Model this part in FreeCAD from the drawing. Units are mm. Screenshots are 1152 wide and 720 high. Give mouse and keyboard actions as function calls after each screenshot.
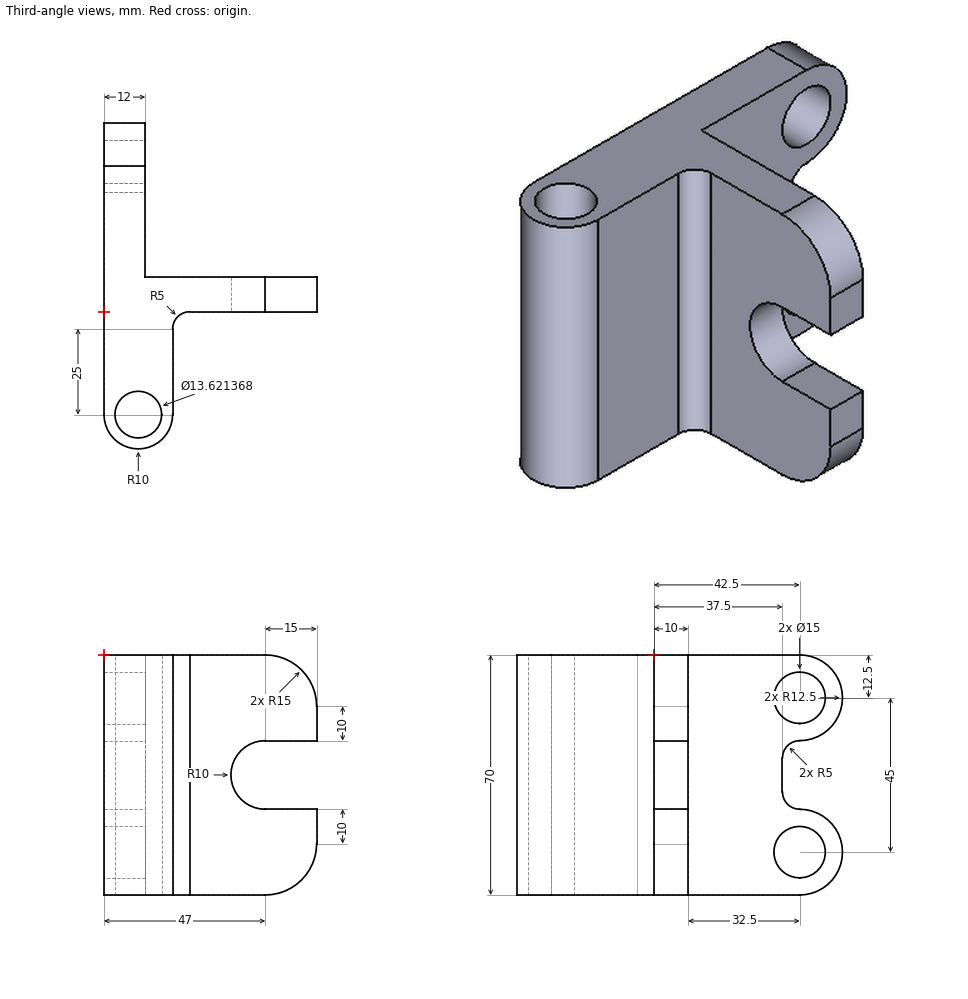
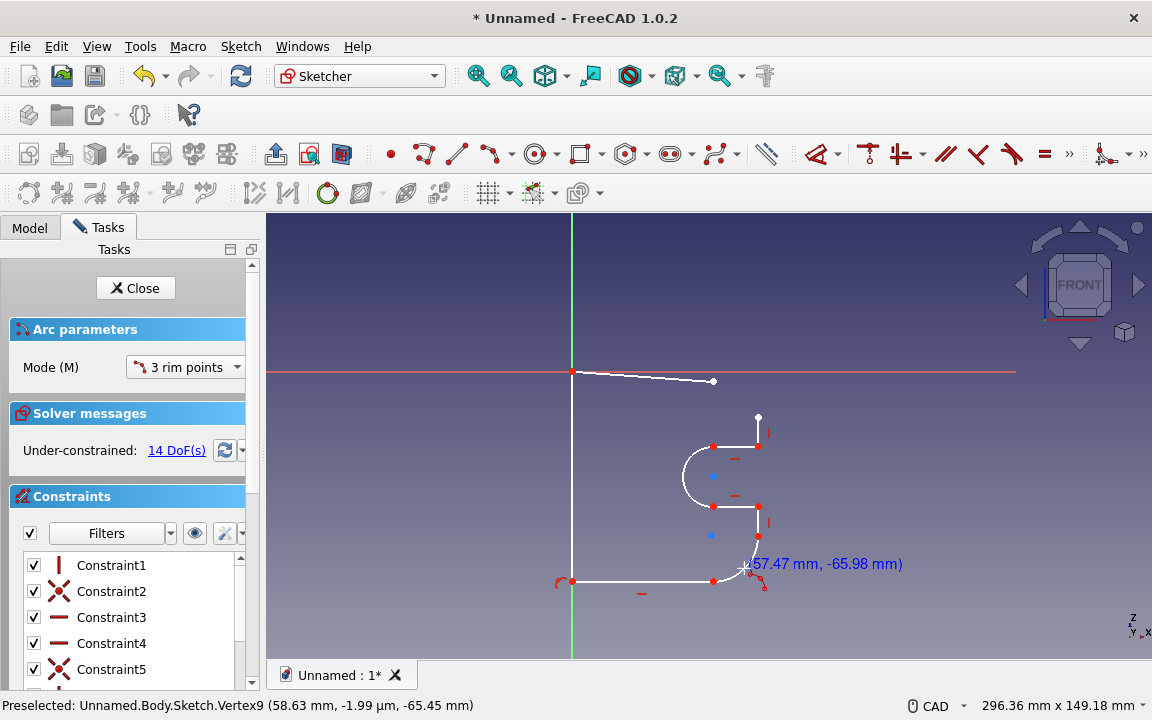
click(713, 382)
click(758, 418)
click(744, 385)
key(Escape)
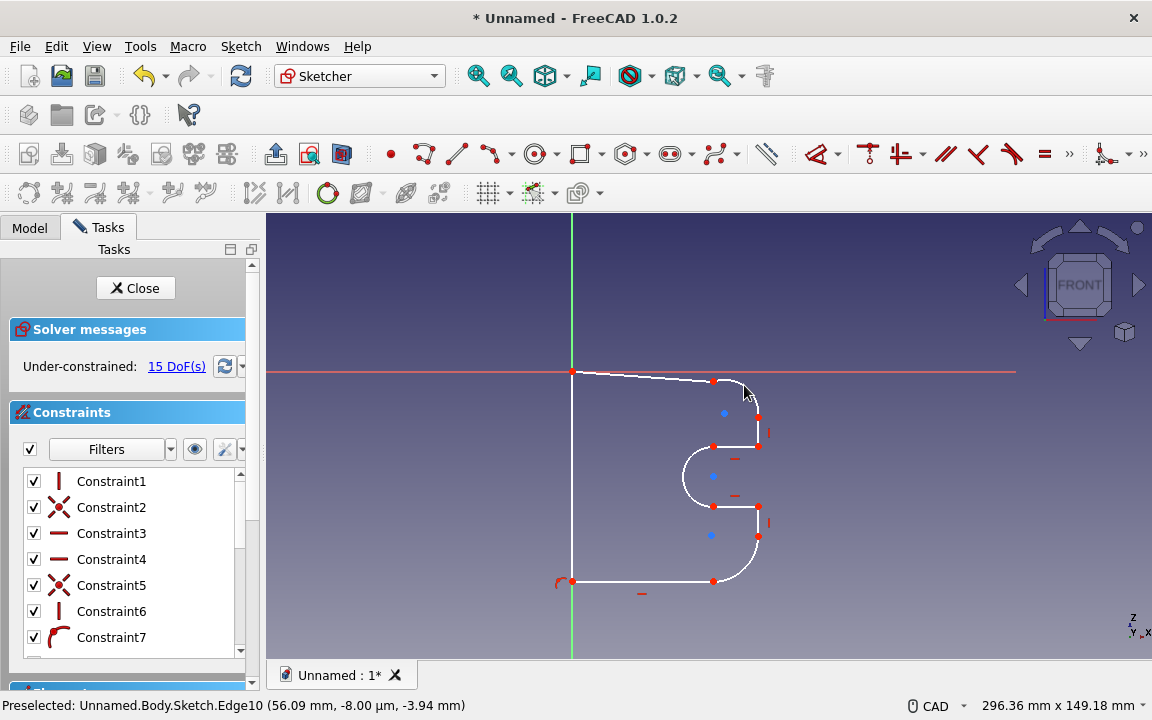
click(758, 430)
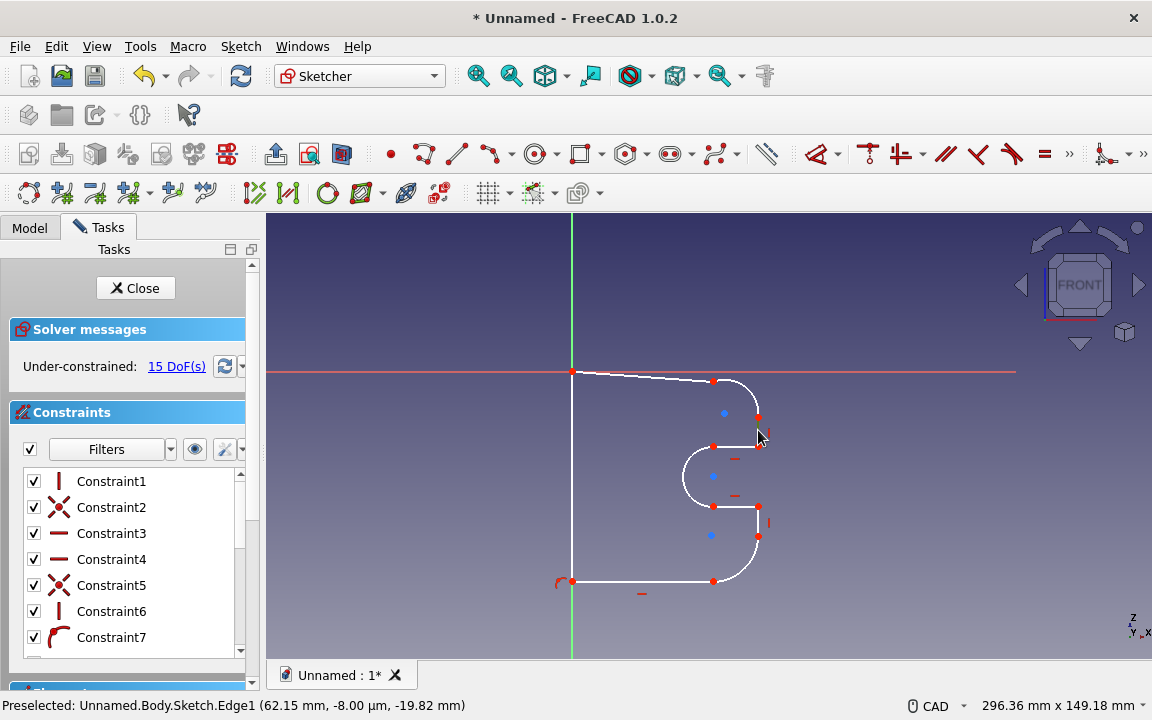
click(754, 398)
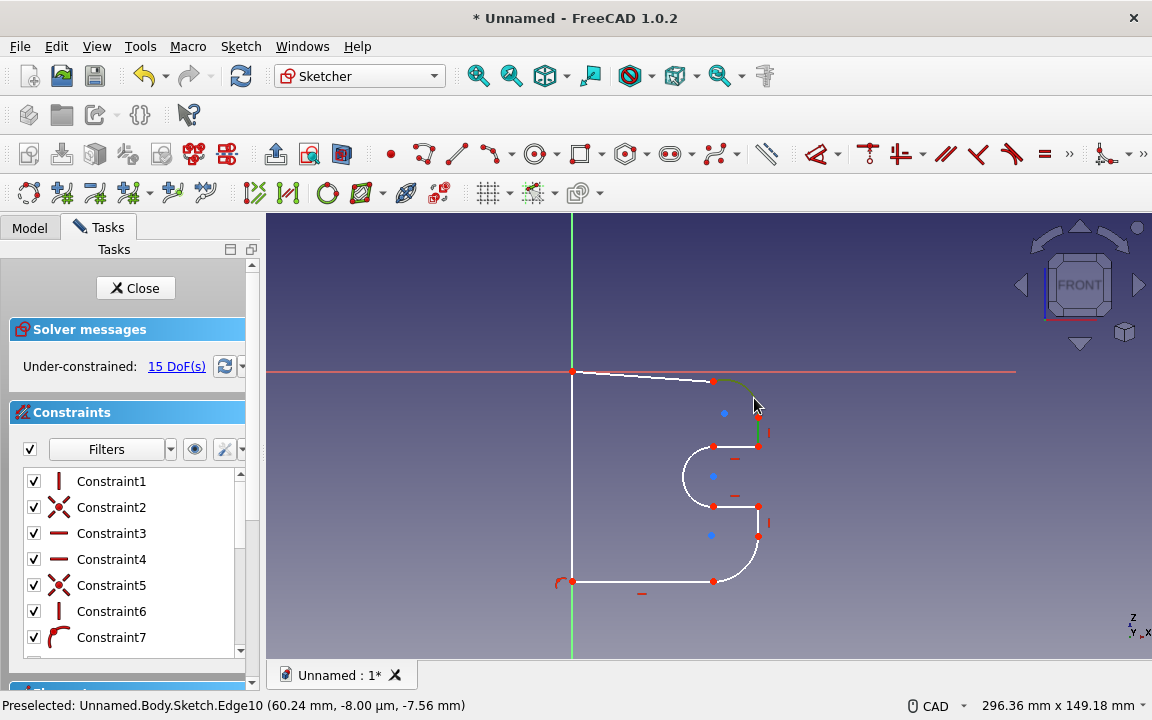
key(t)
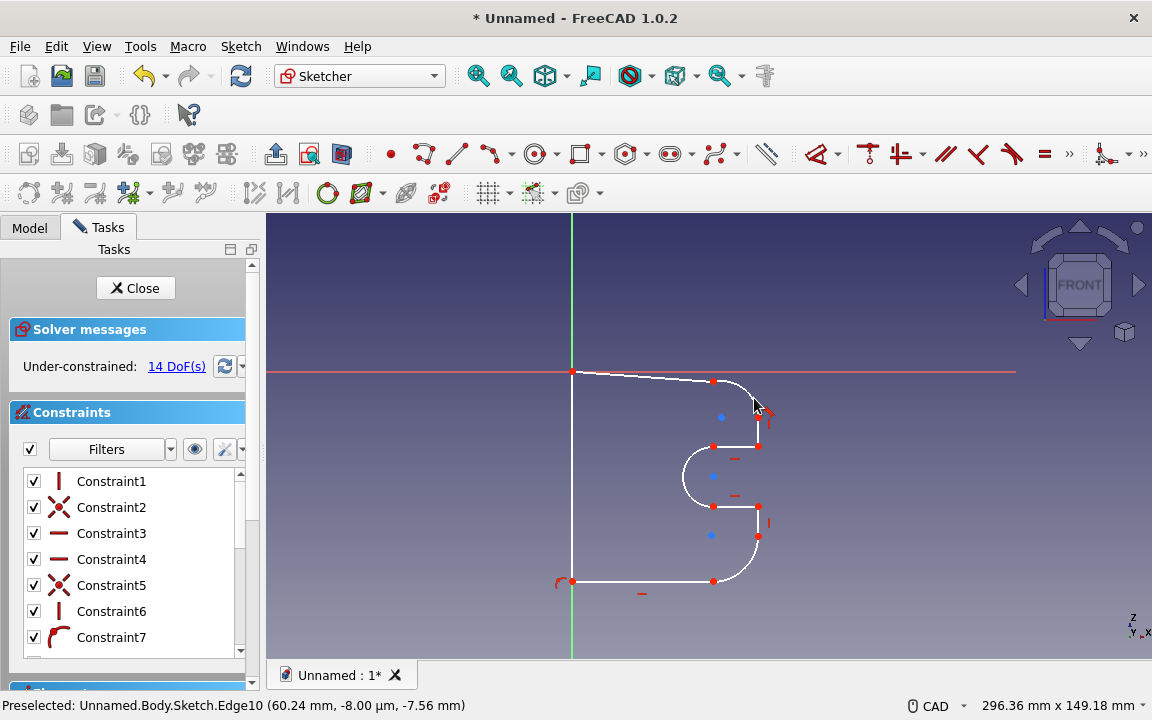
click(745, 447)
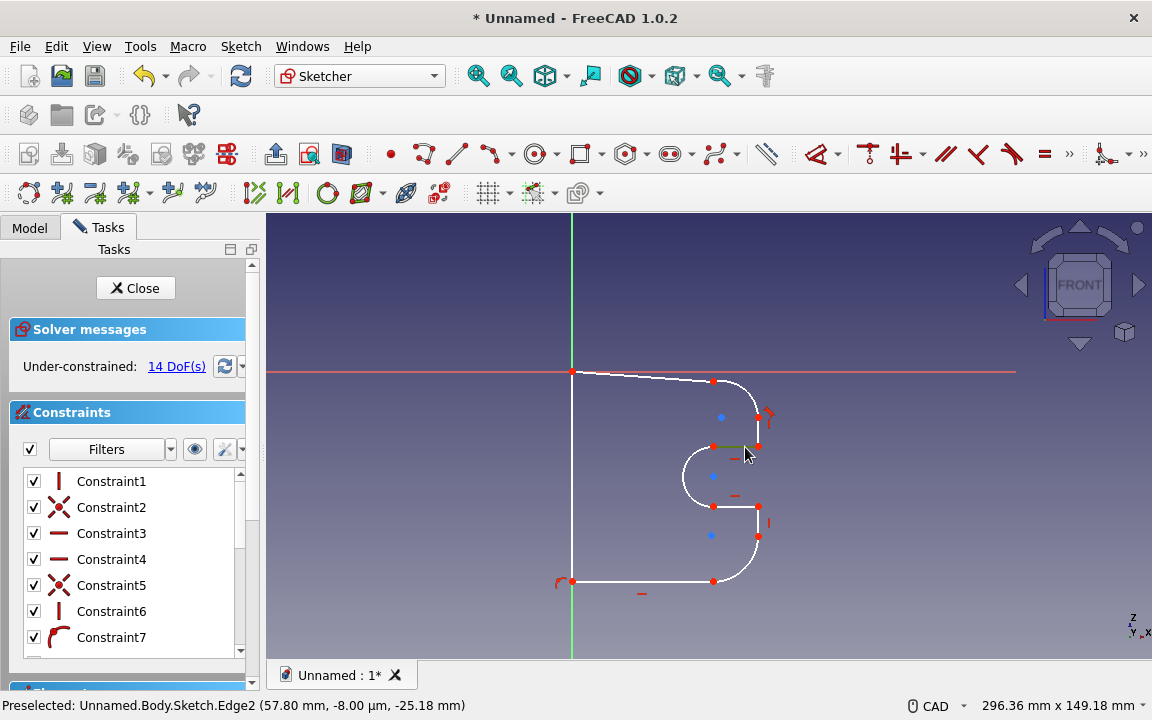
click(689, 459)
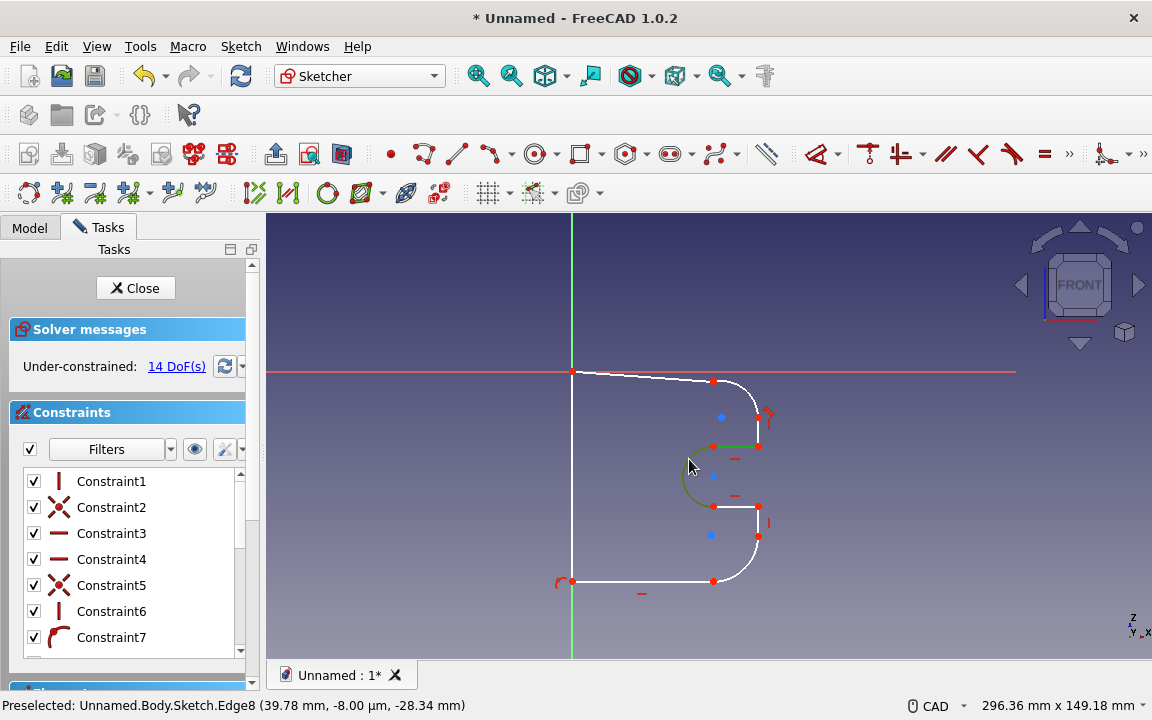
click(1012, 154)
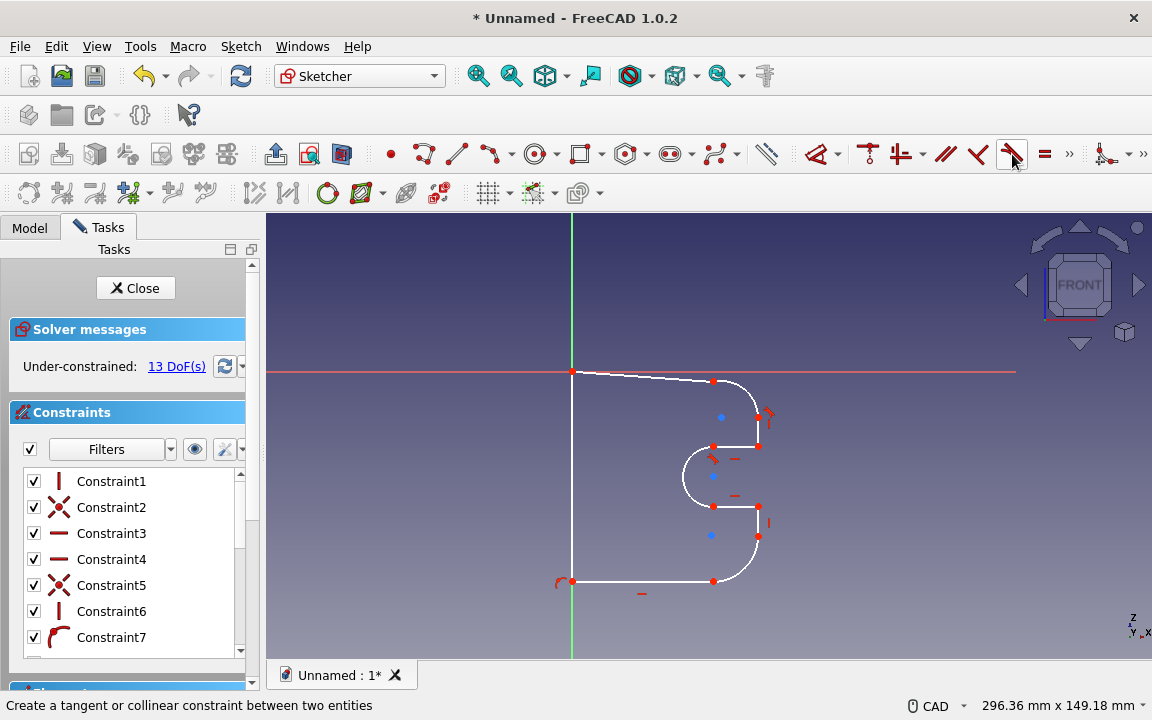
click(727, 507)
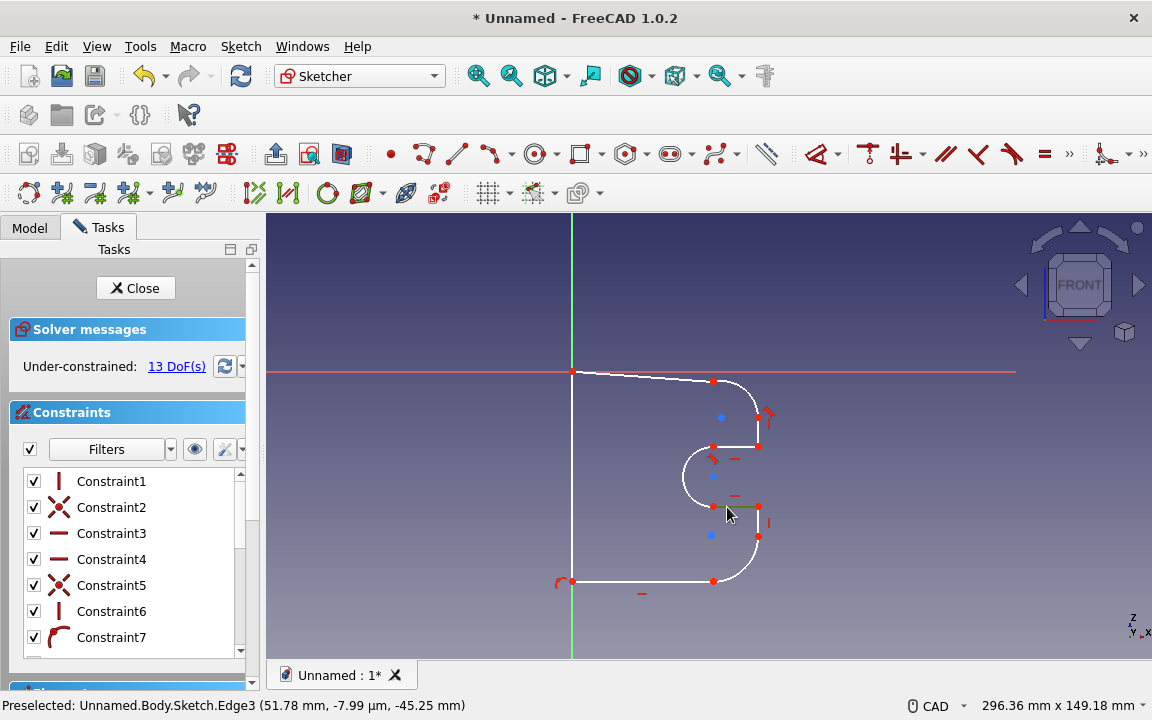
click(689, 459)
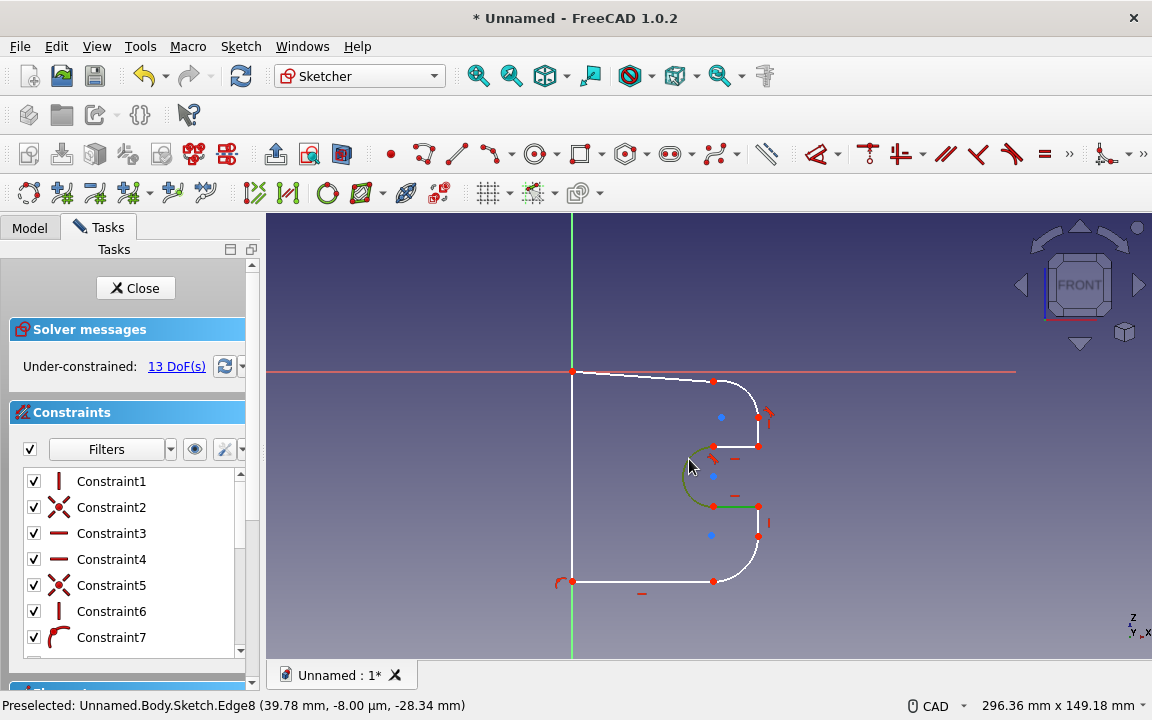
key(t)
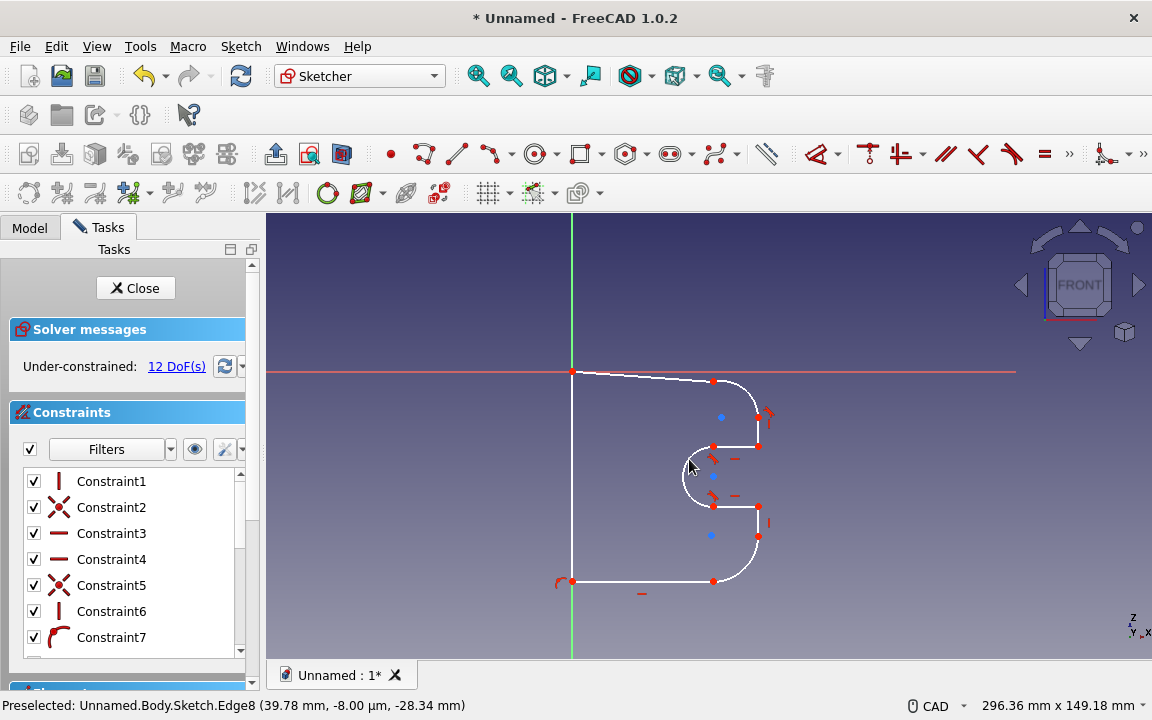
click(758, 519)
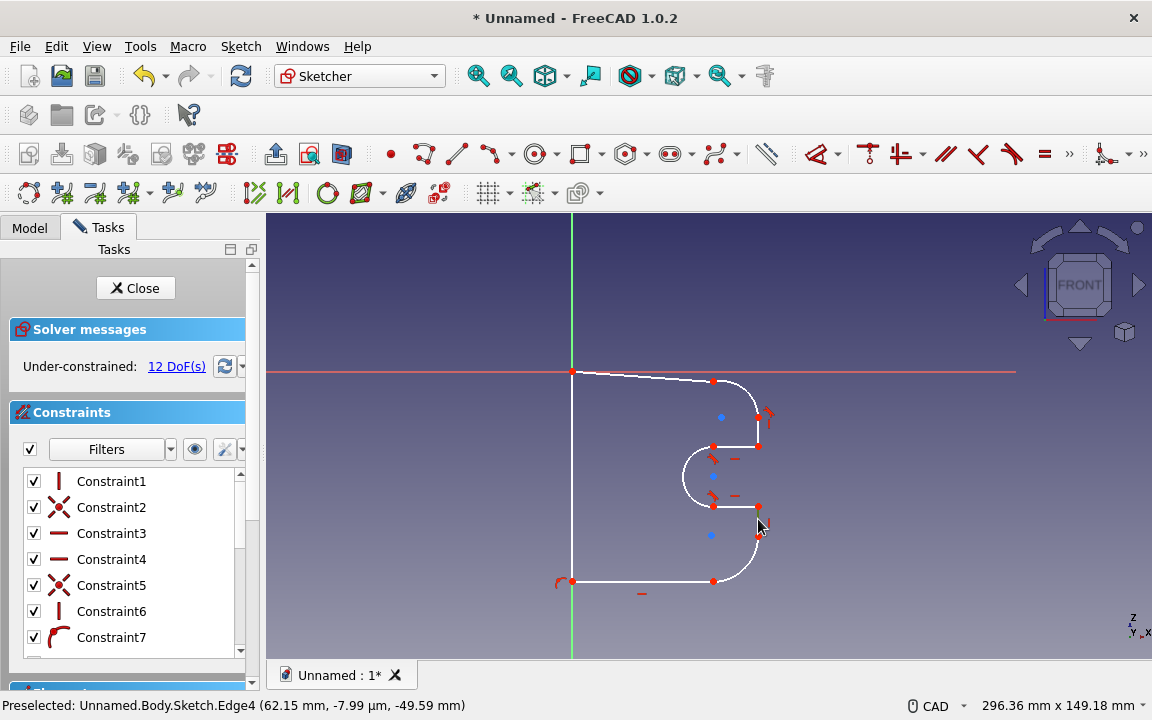
click(733, 577)